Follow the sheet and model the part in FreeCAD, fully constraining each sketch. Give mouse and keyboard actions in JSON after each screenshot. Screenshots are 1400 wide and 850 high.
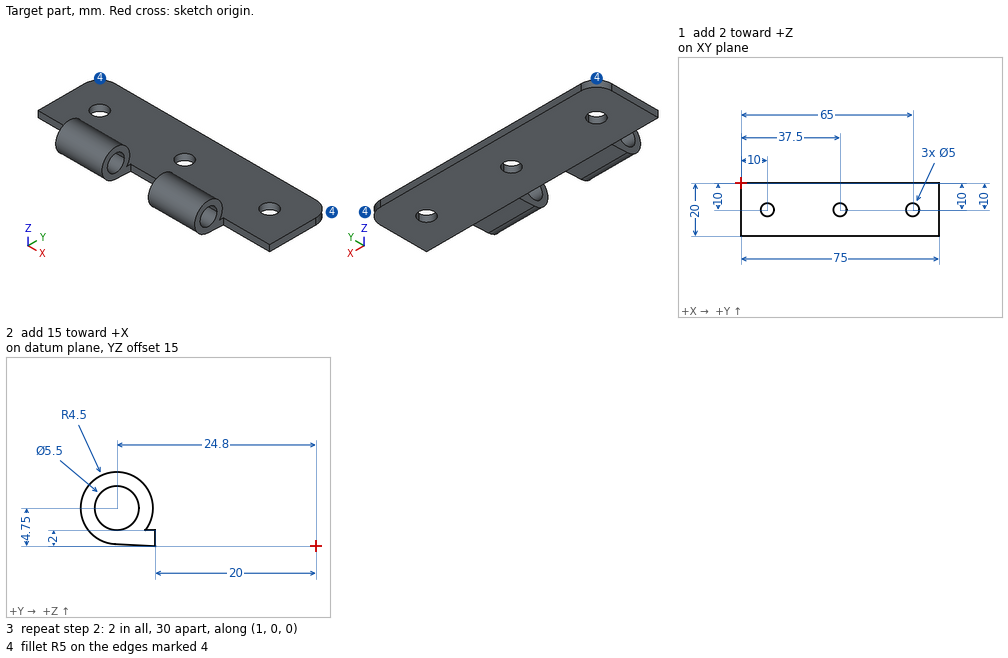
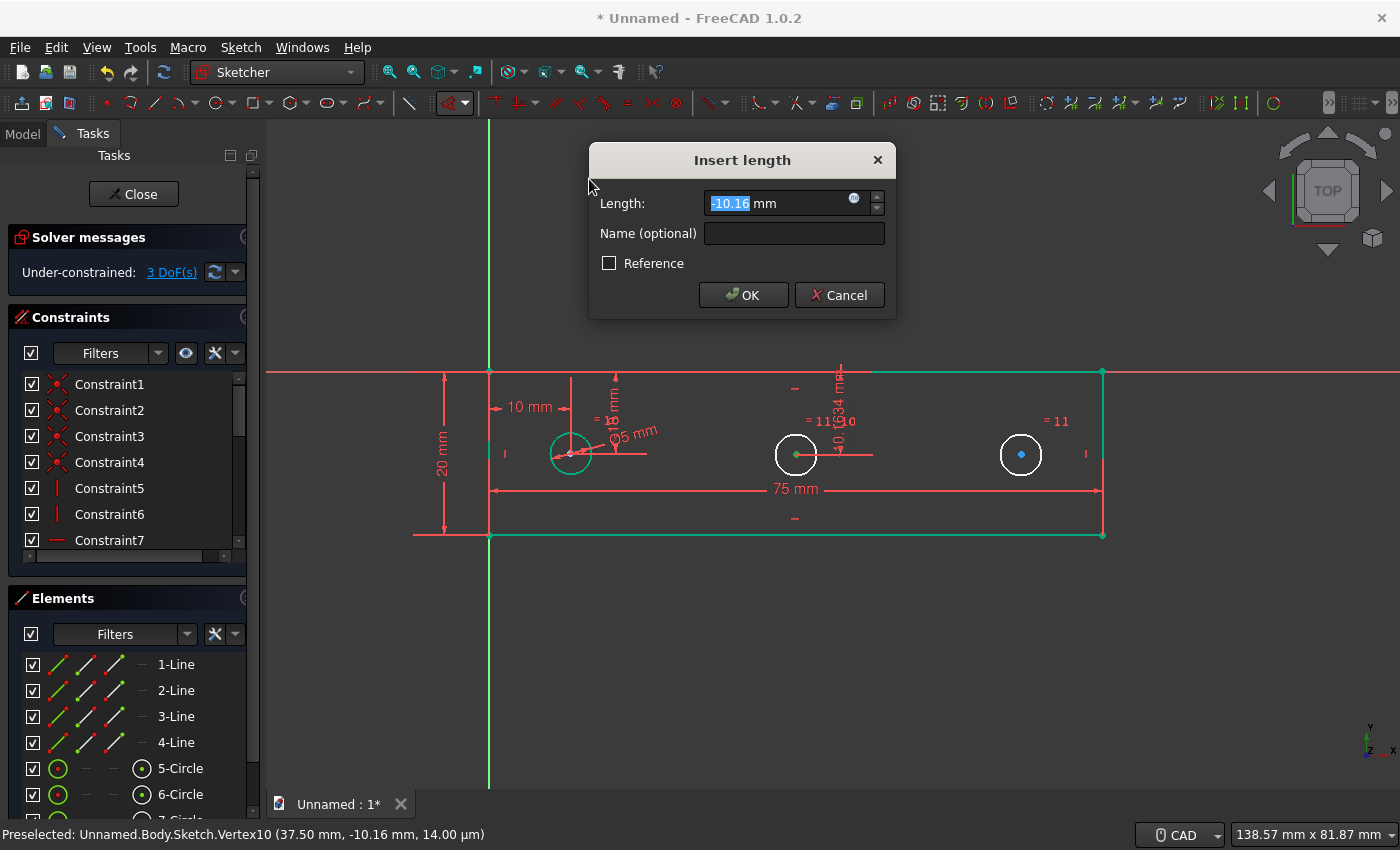
{"action": "type", "text": "-10"}
{"action": "key", "text": "Return"}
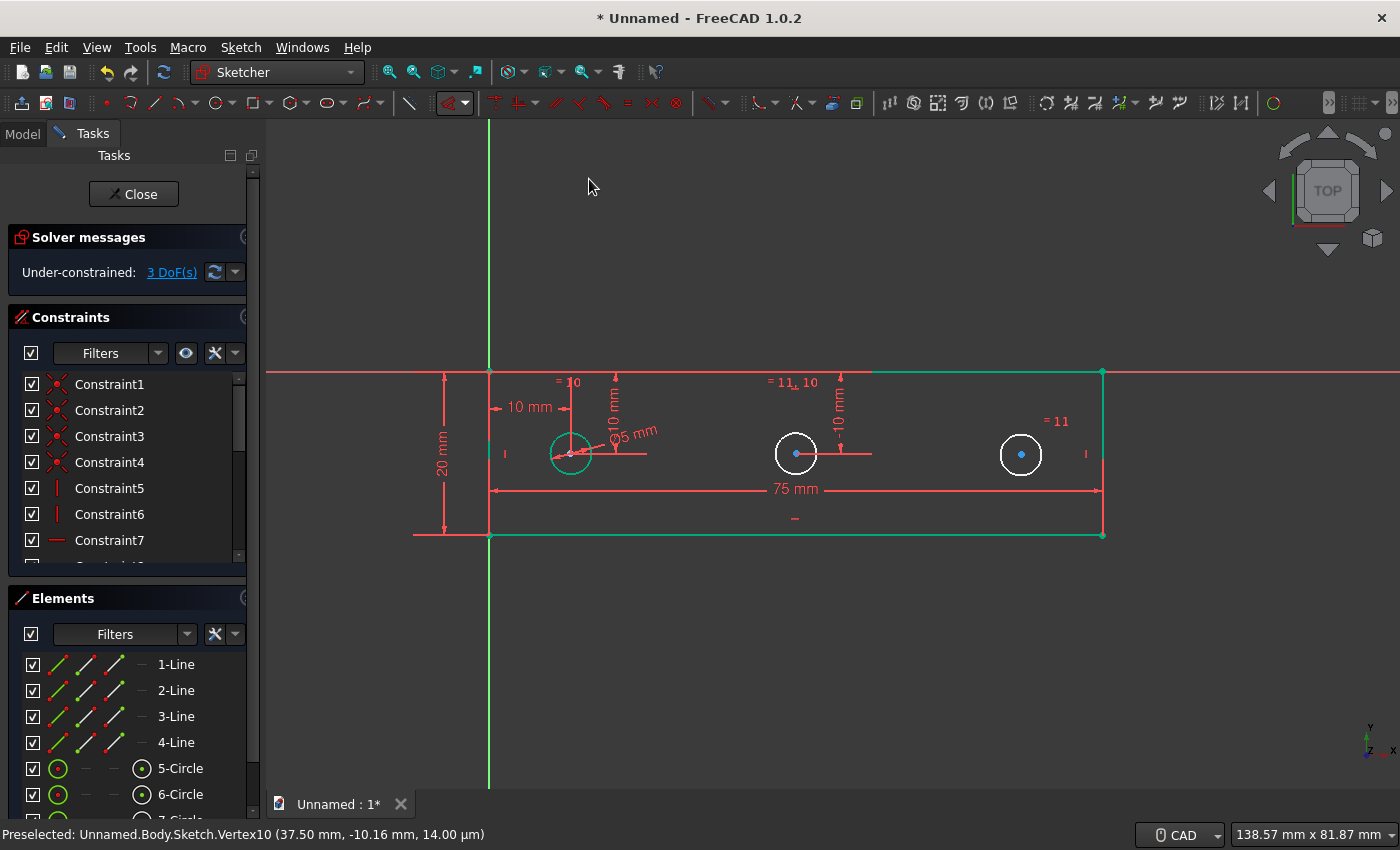
{"action": "left_click", "coordinate": [1021, 455]}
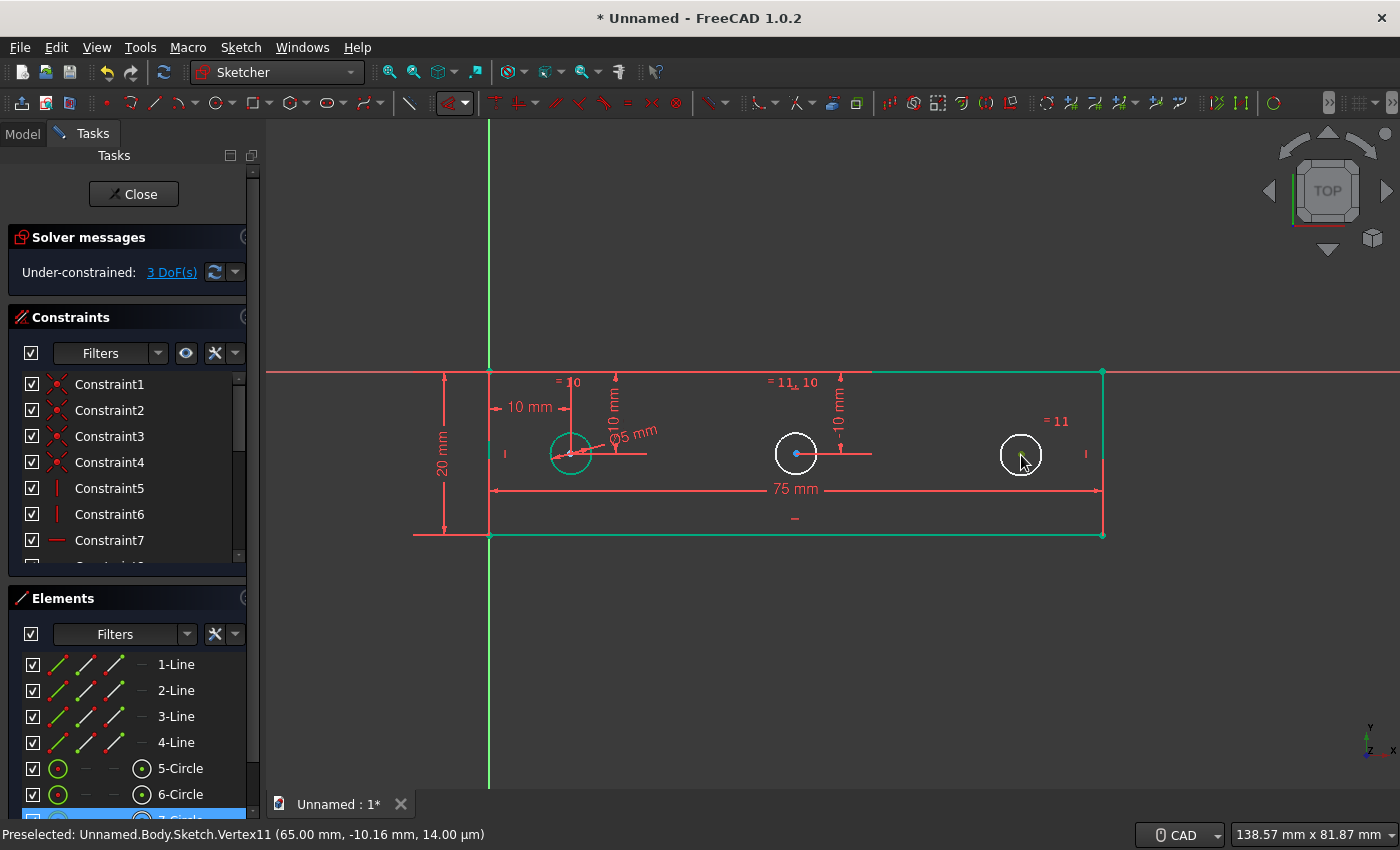
{"action": "key", "text": "l"}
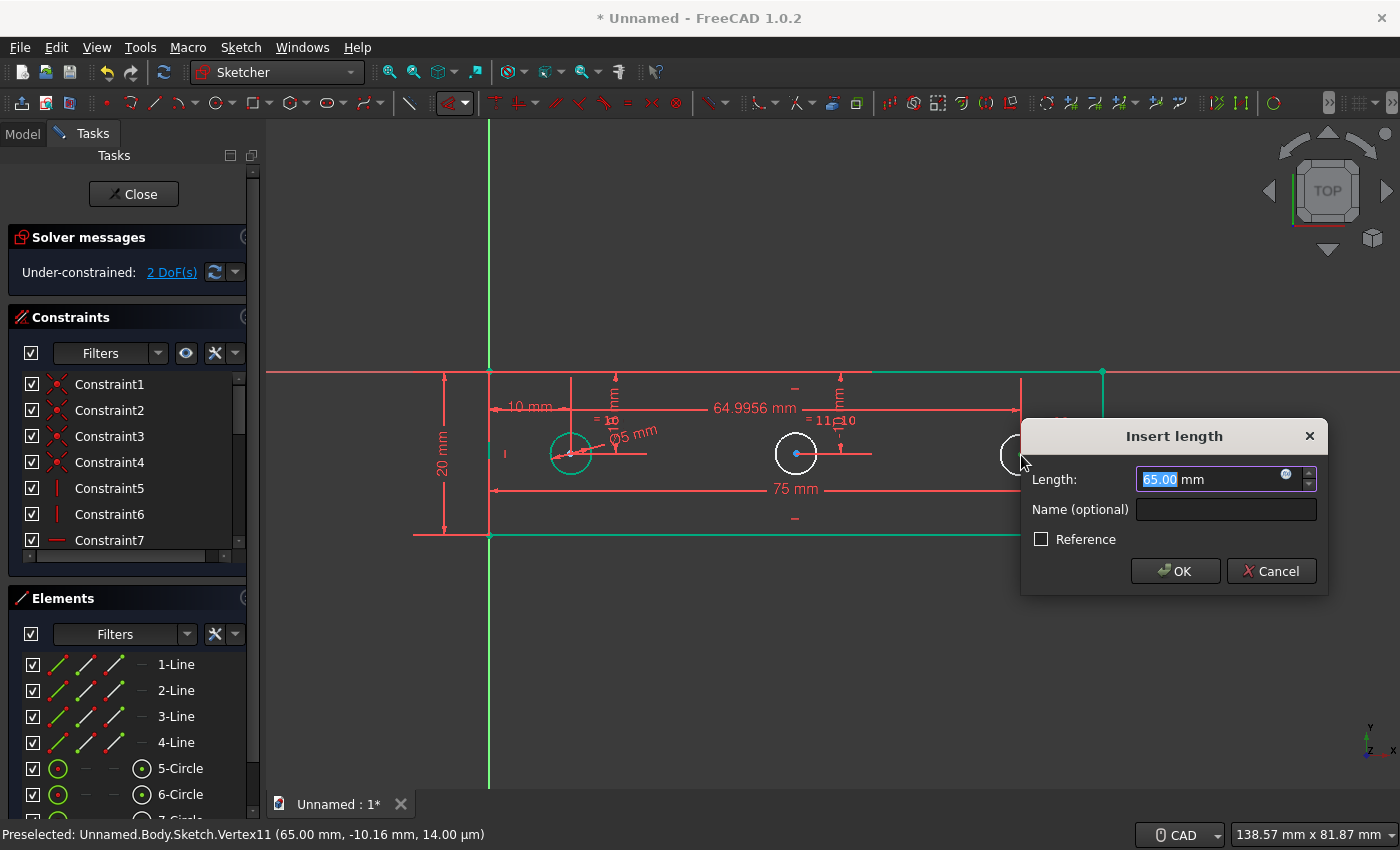
{"action": "type", "text": "65"}
{"action": "key", "text": "Return"}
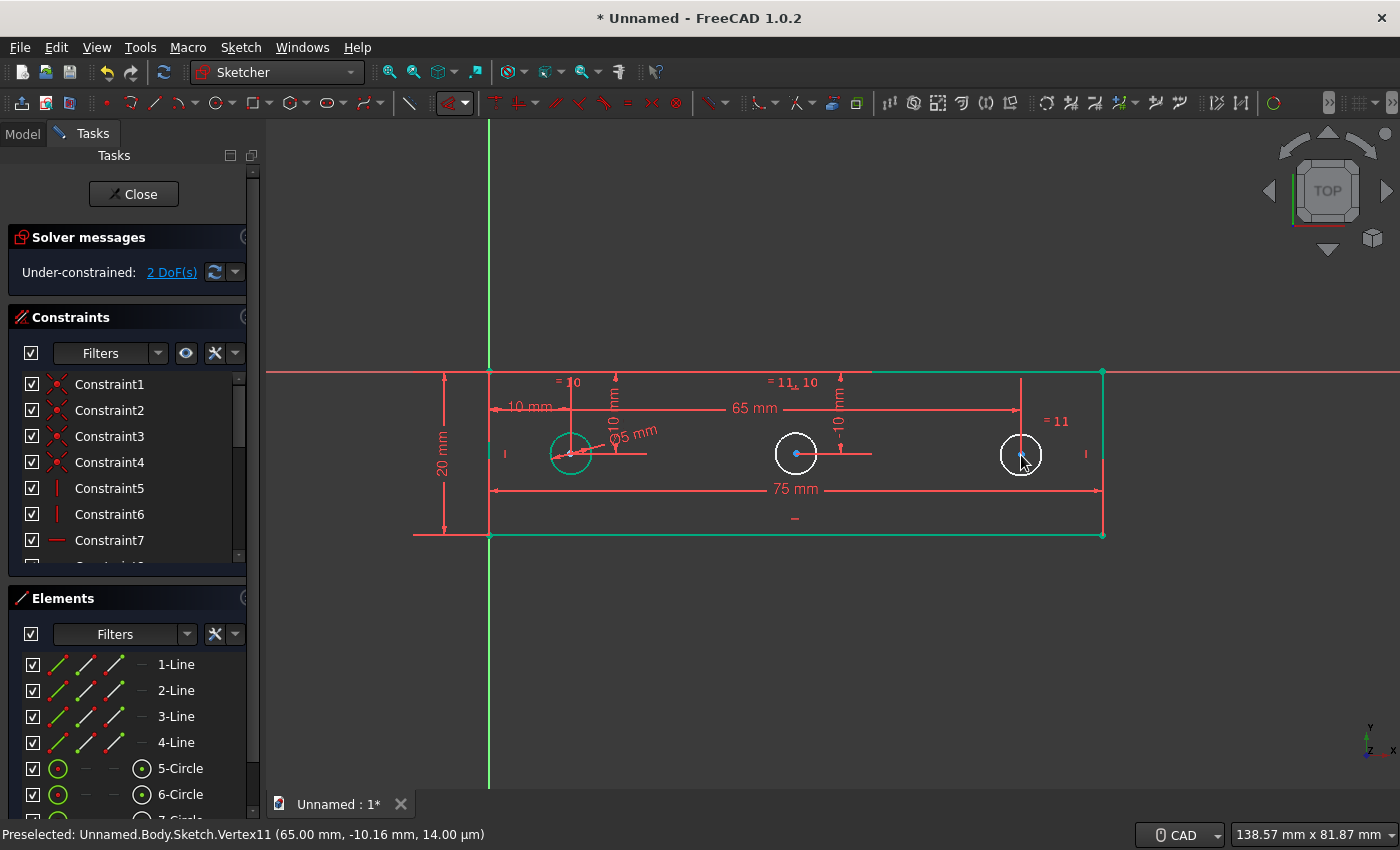
{"action": "left_click", "coordinate": [1021, 455]}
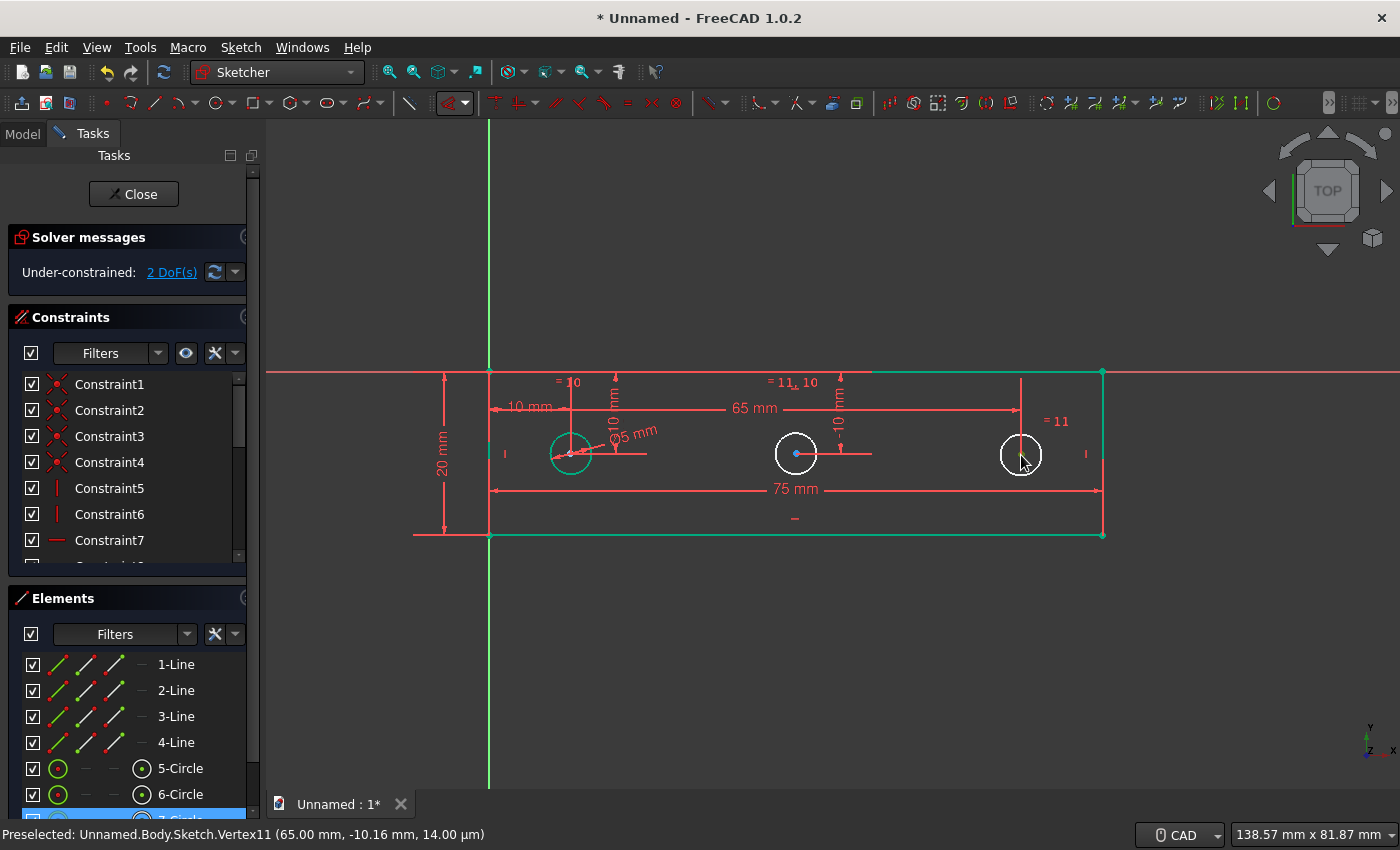
{"action": "key", "text": "i"}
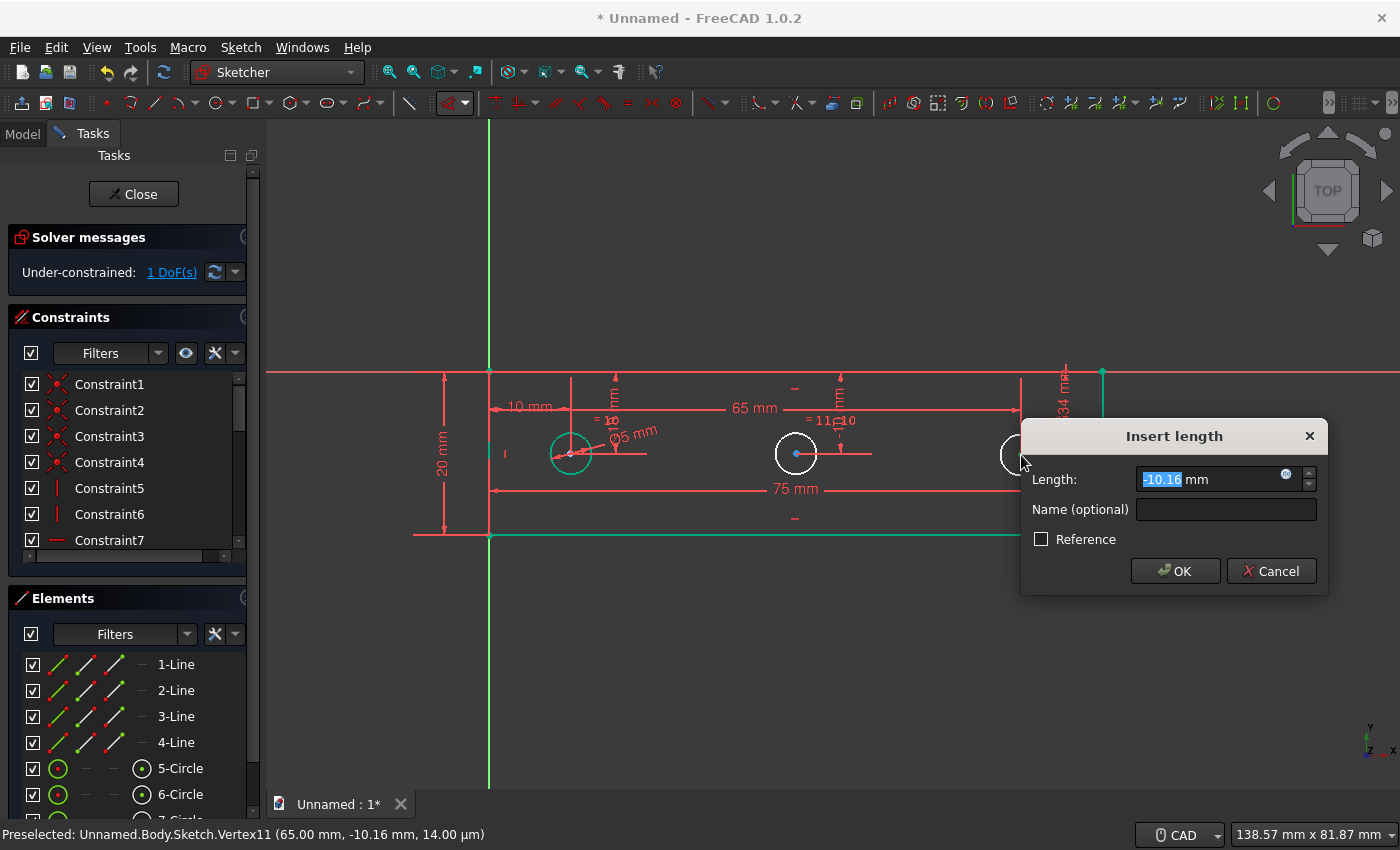
{"action": "type", "text": "-10"}
{"action": "key", "text": "Return"}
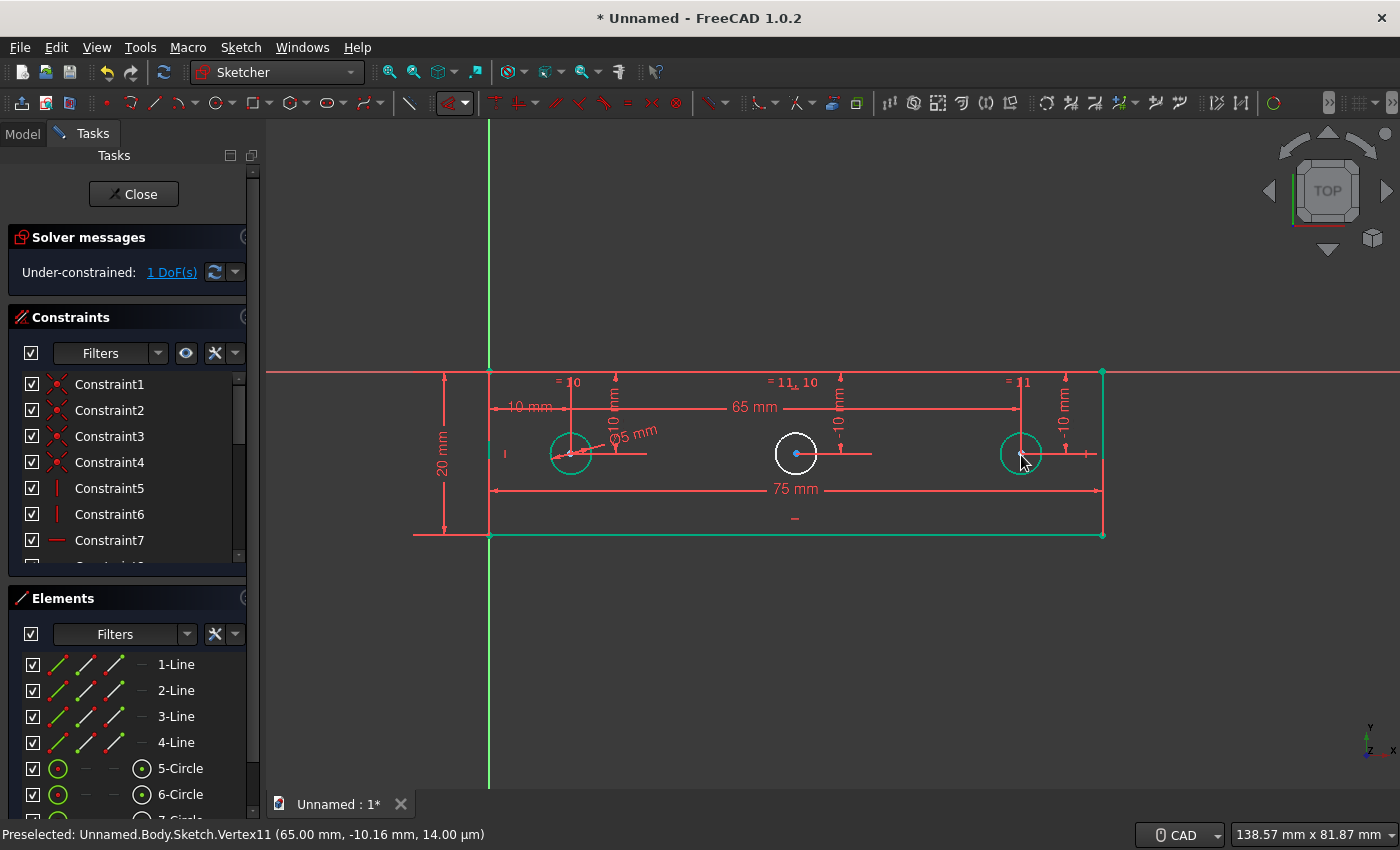
{"action": "left_click", "coordinate": [796, 454]}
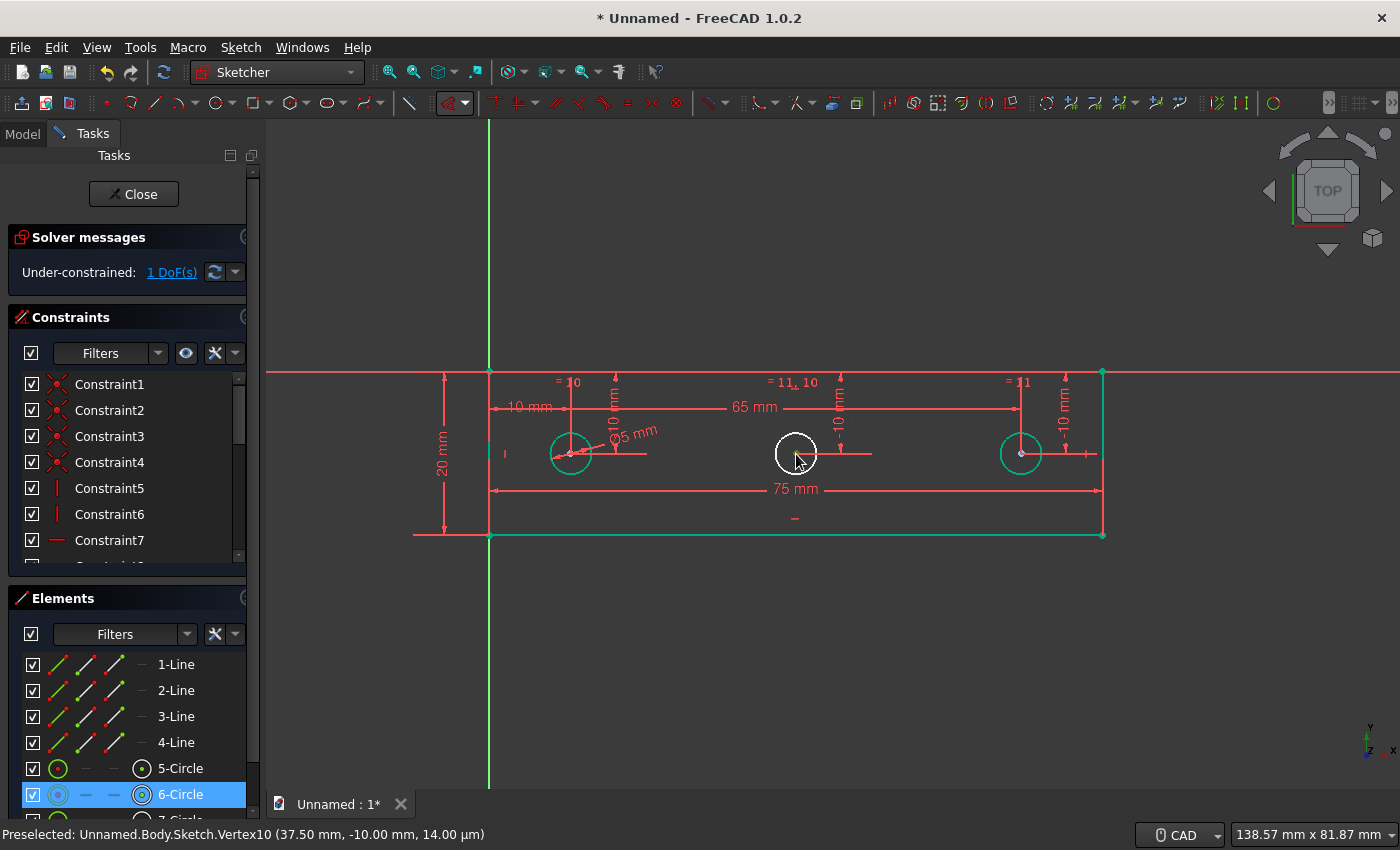
{"action": "key", "text": "l"}